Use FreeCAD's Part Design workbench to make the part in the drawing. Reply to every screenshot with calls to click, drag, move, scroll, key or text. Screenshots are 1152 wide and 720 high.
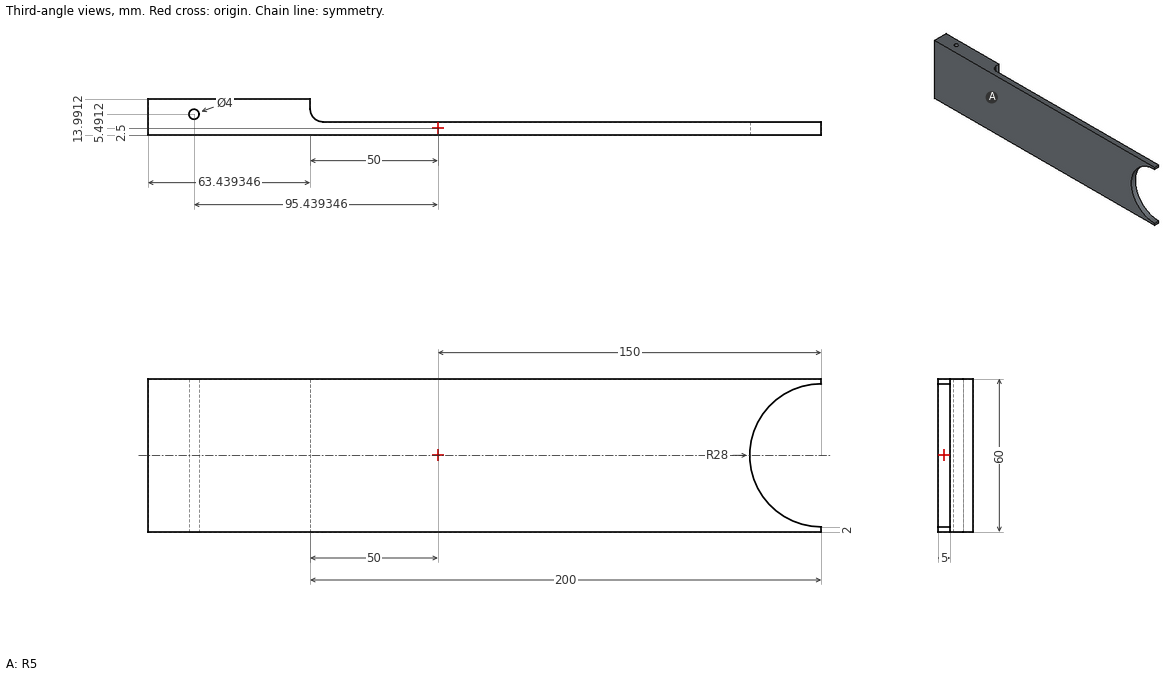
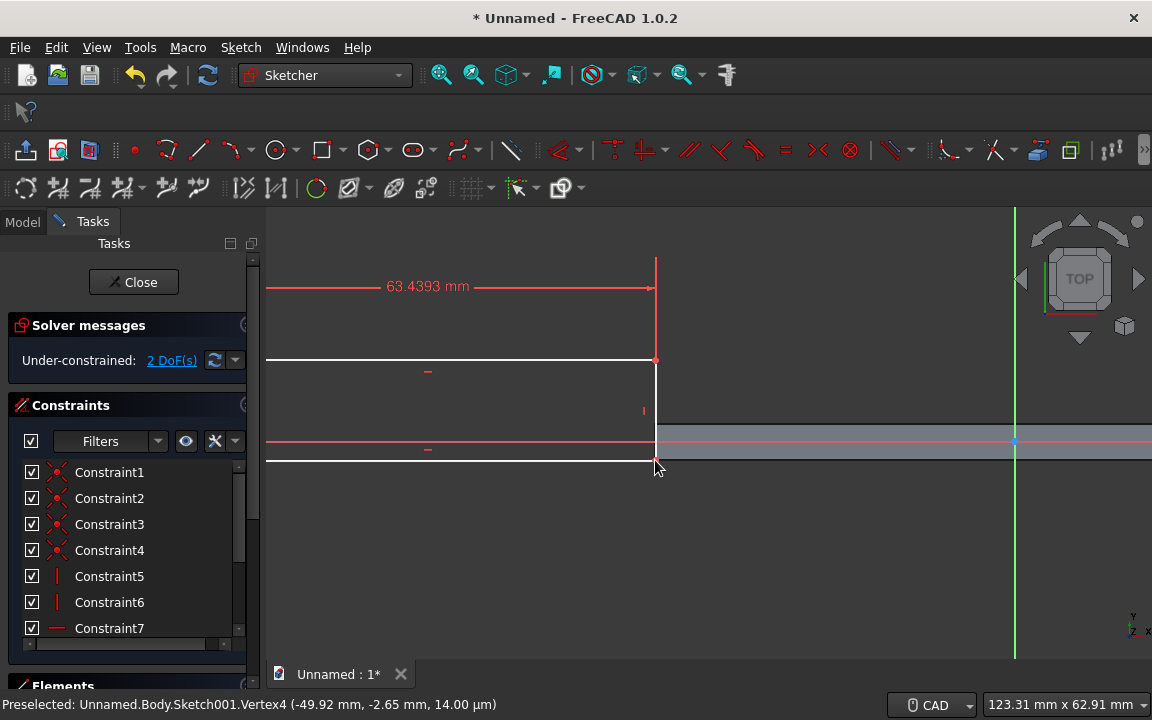
key(d)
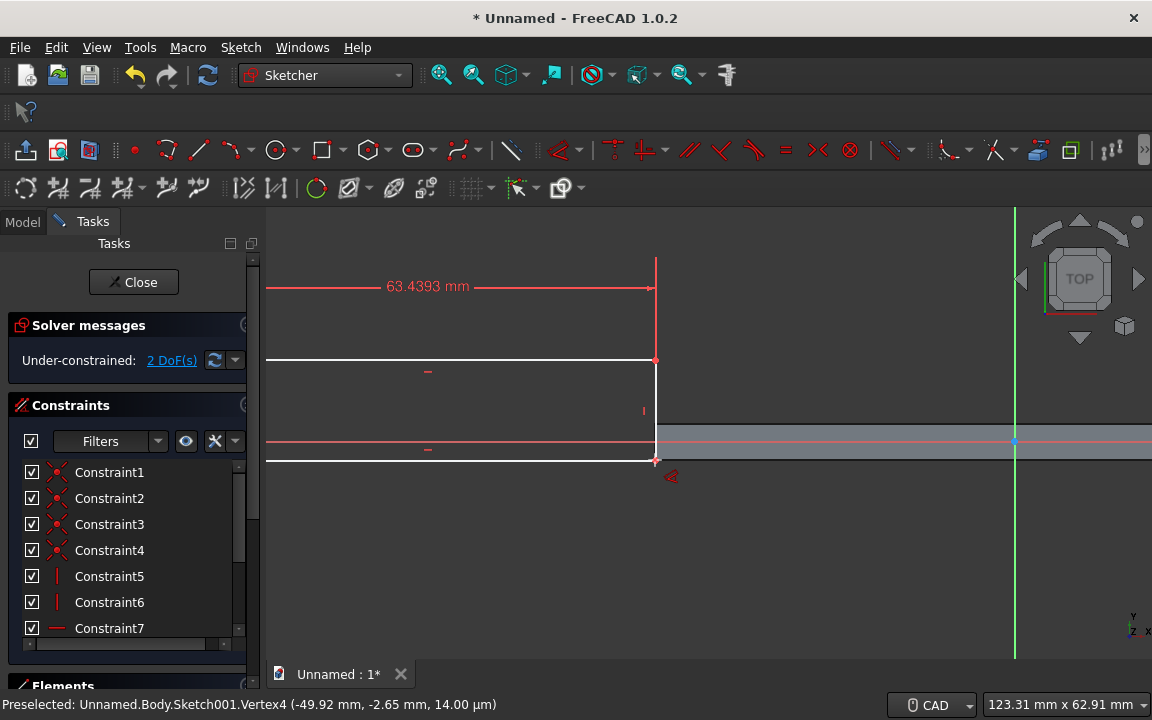
click(656, 461)
click(821, 495)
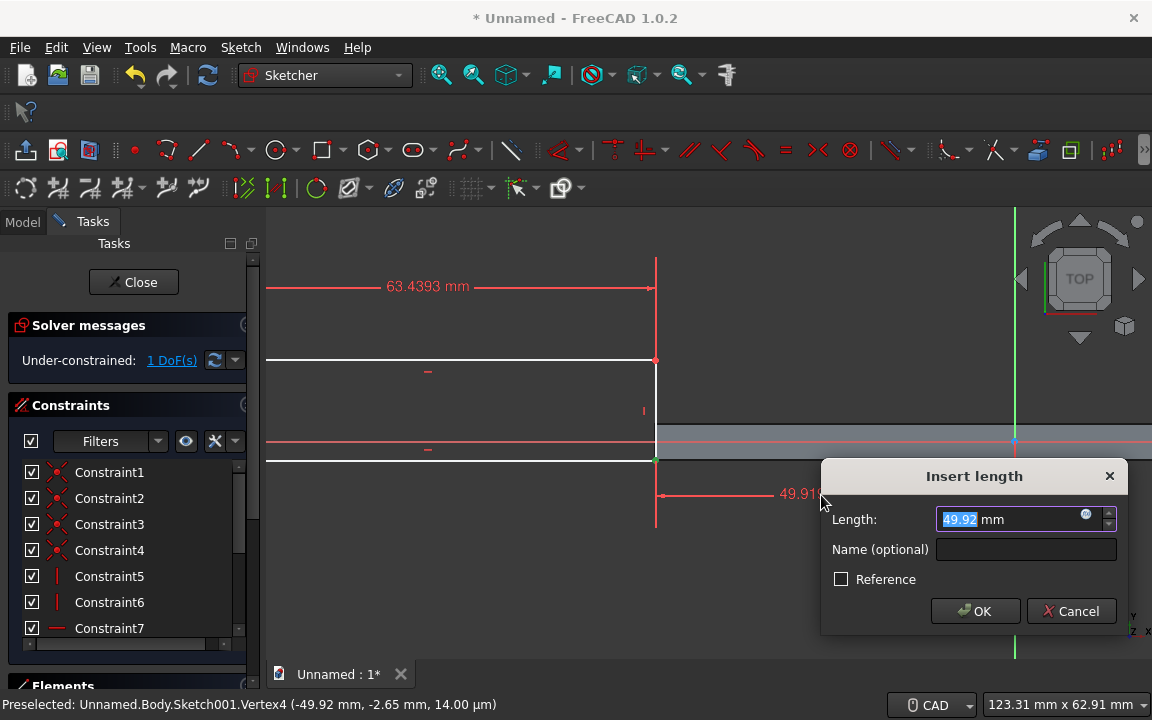
text(50)
key(Return)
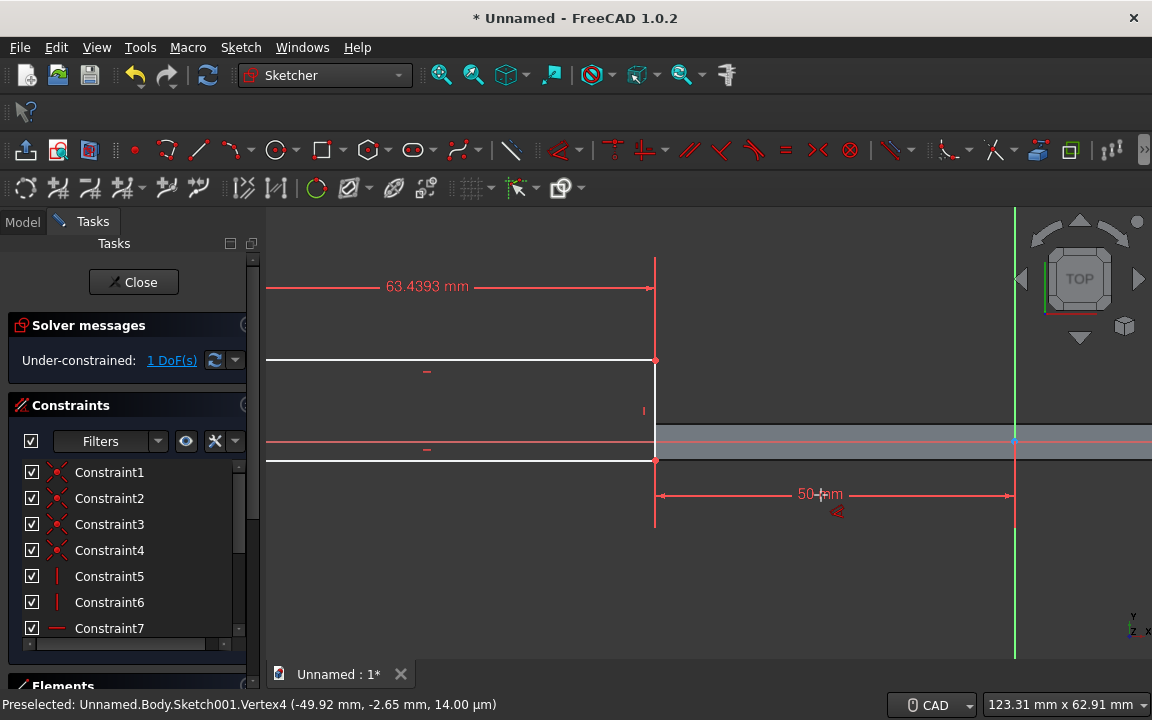
scroll(681, 462, down, 3)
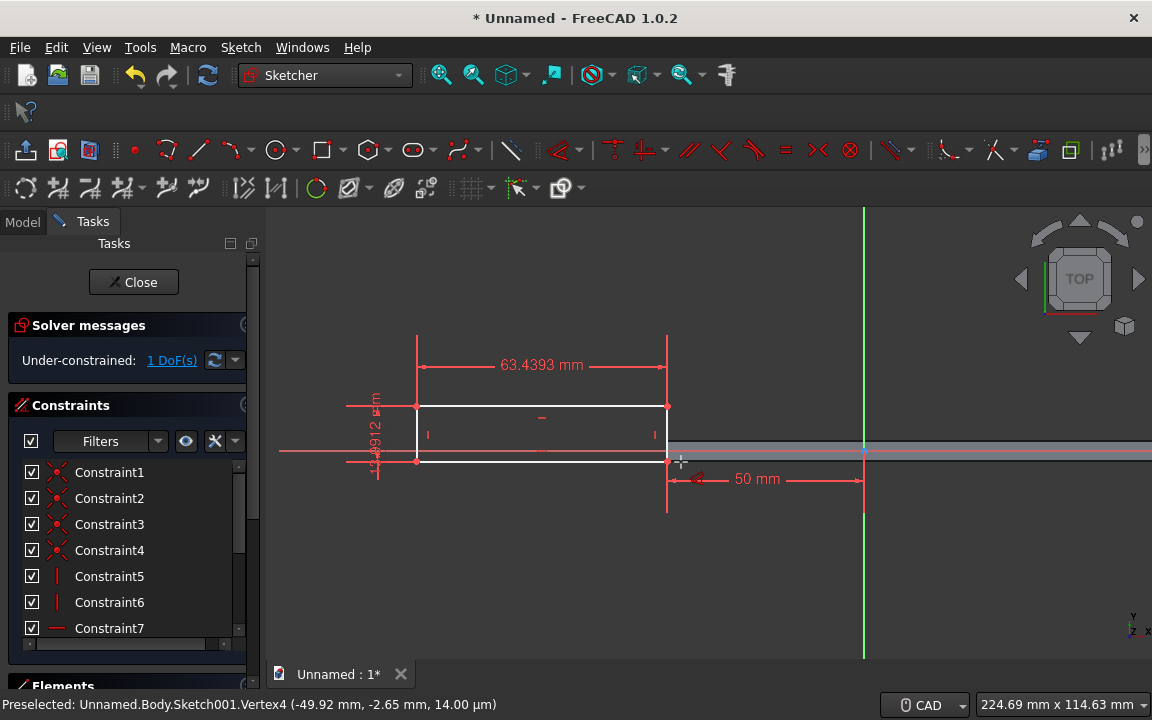
scroll(417, 462, up, 7)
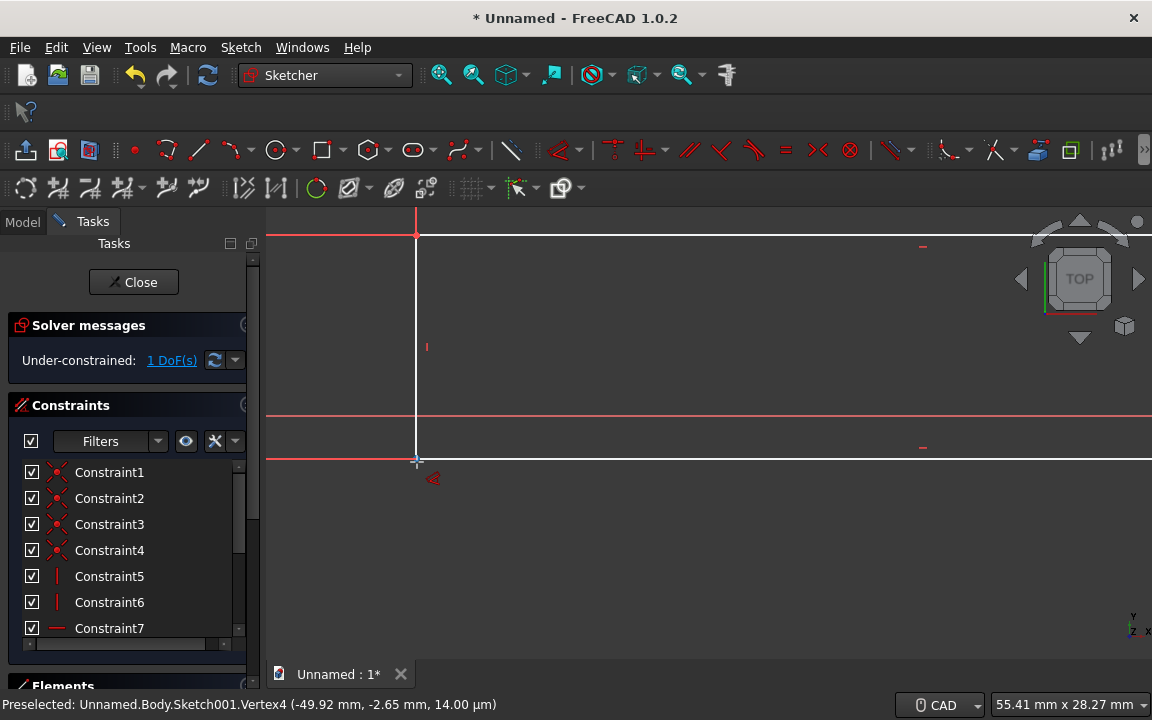
click(416, 459)
click(382, 438)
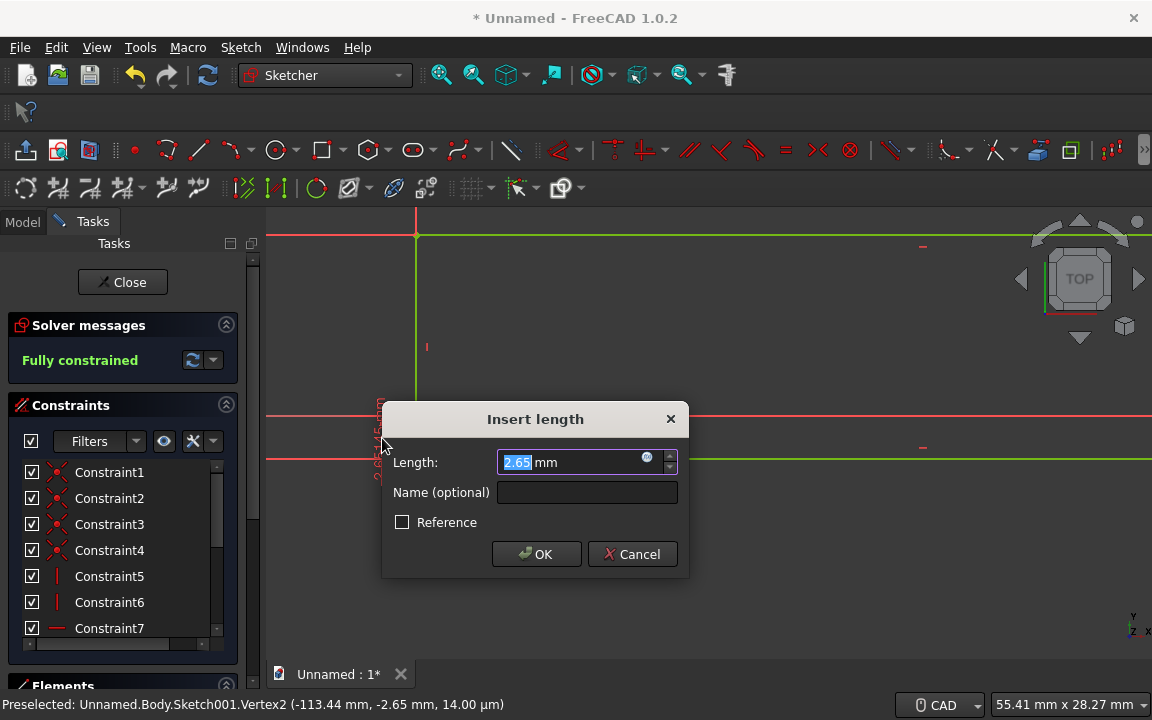
text(2.5)
key(Return)
key(Escape)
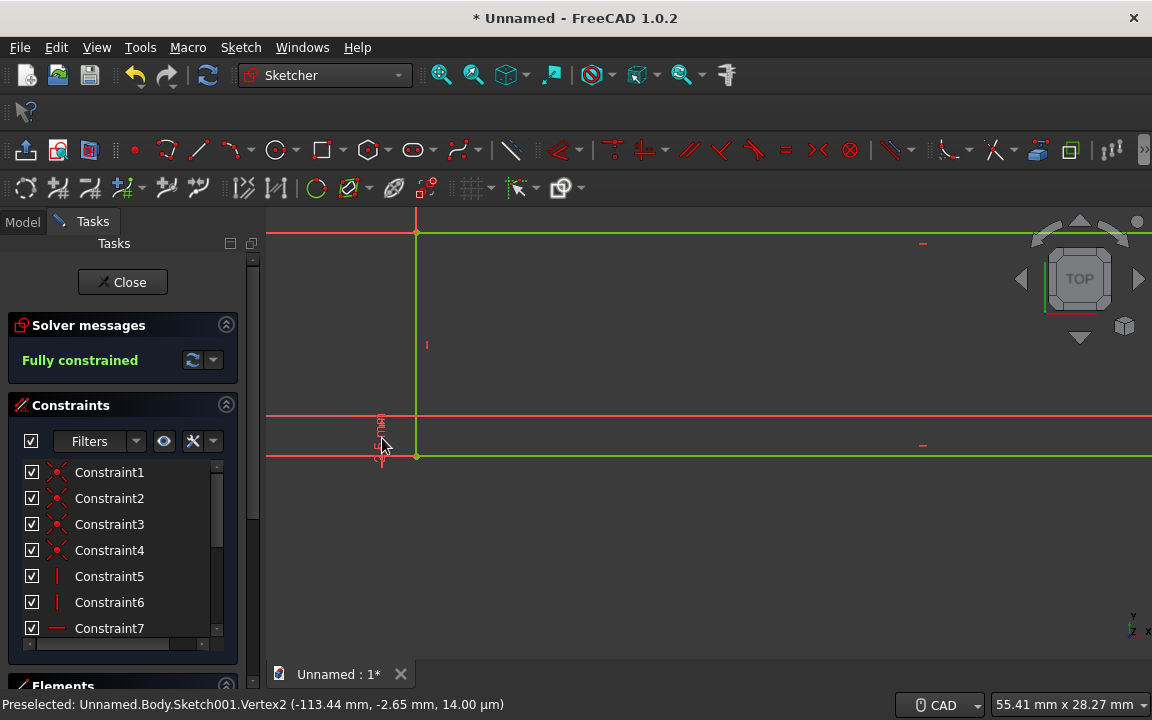
click(123, 282)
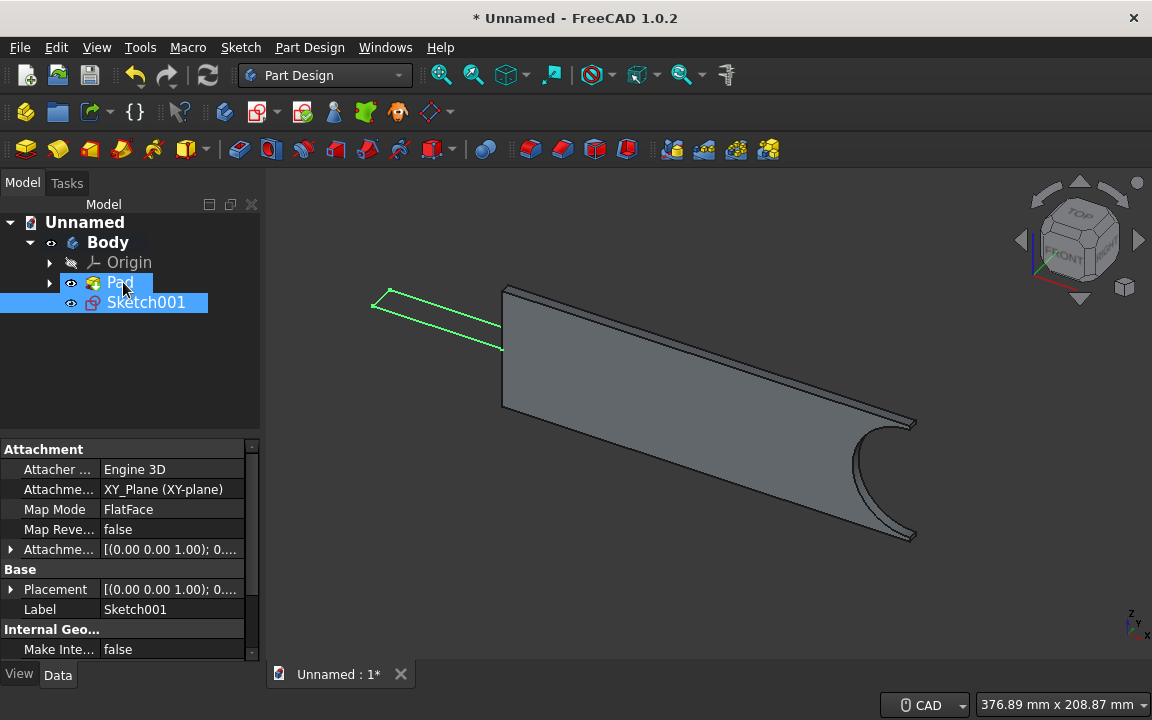
click(26, 150)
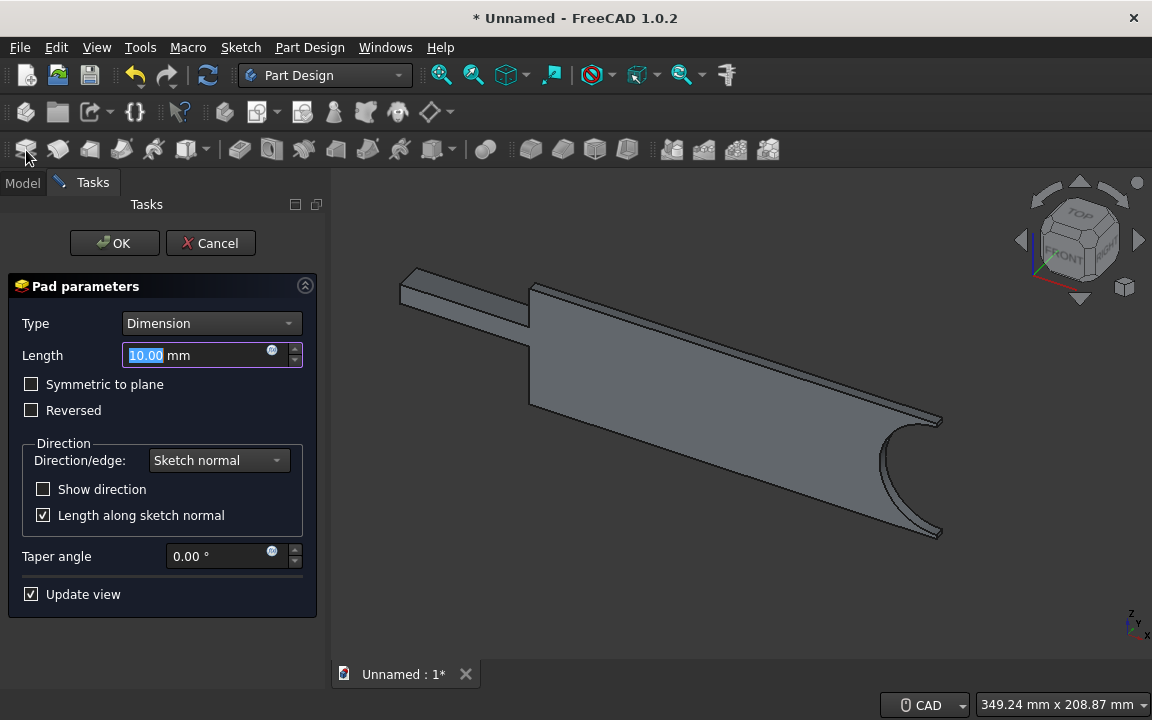
text(60)
key(Tab)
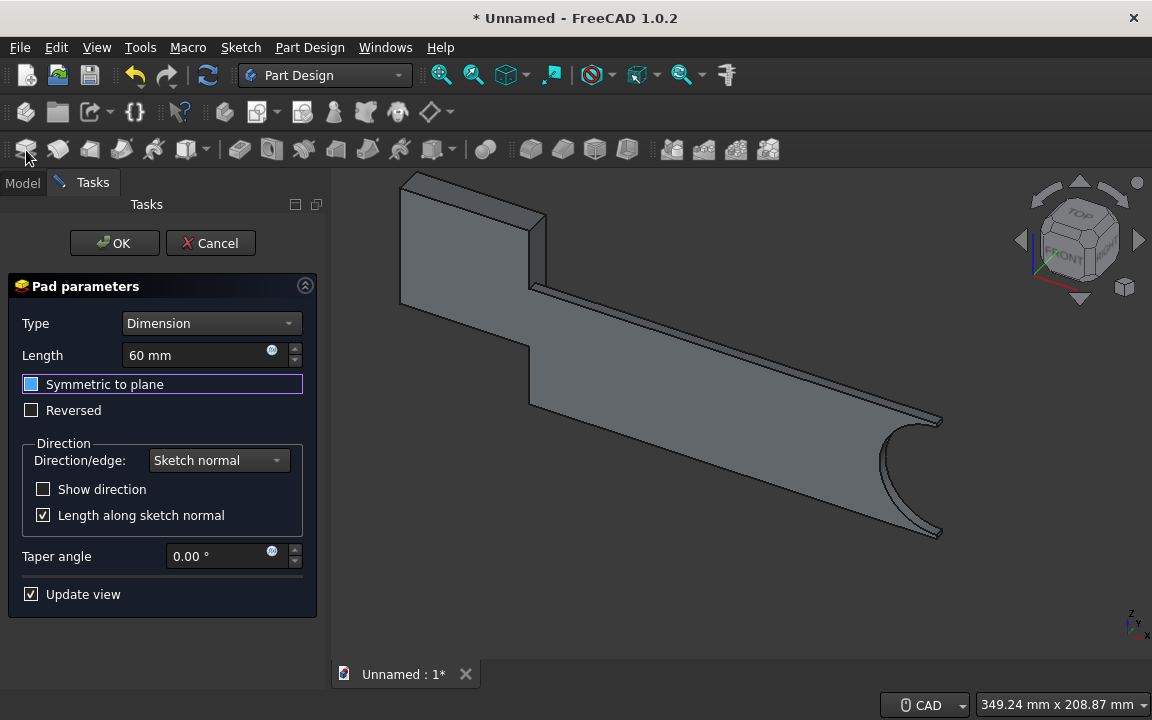
click(30, 384)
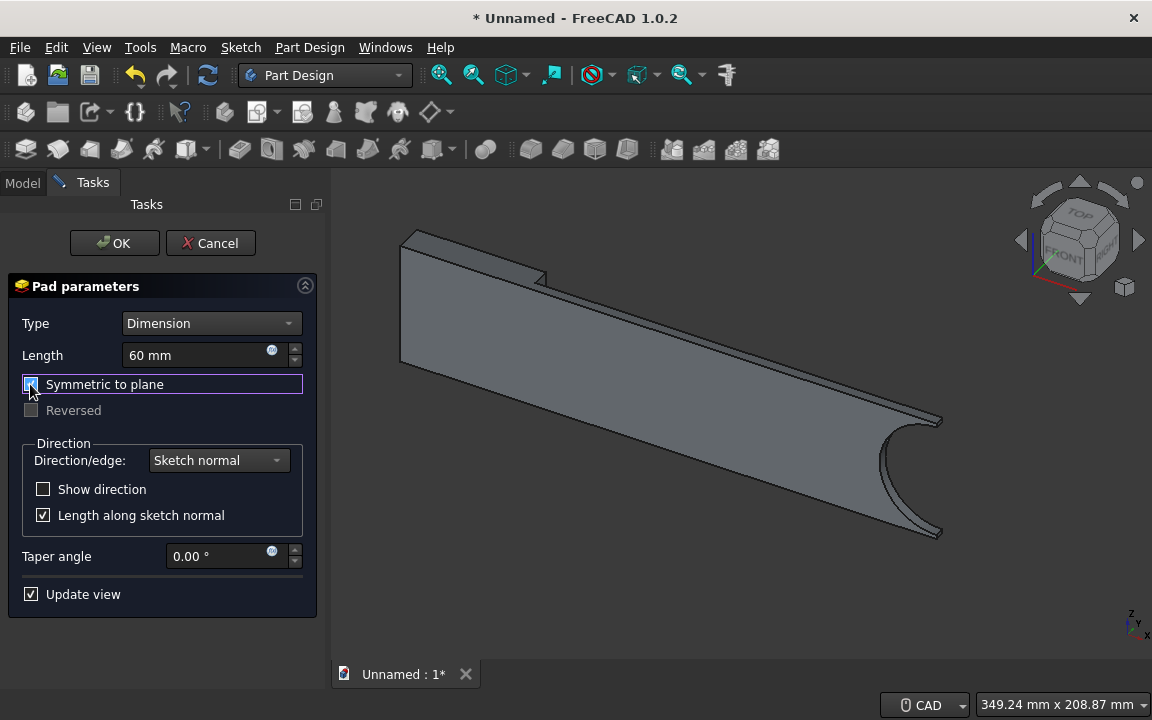
click(115, 243)